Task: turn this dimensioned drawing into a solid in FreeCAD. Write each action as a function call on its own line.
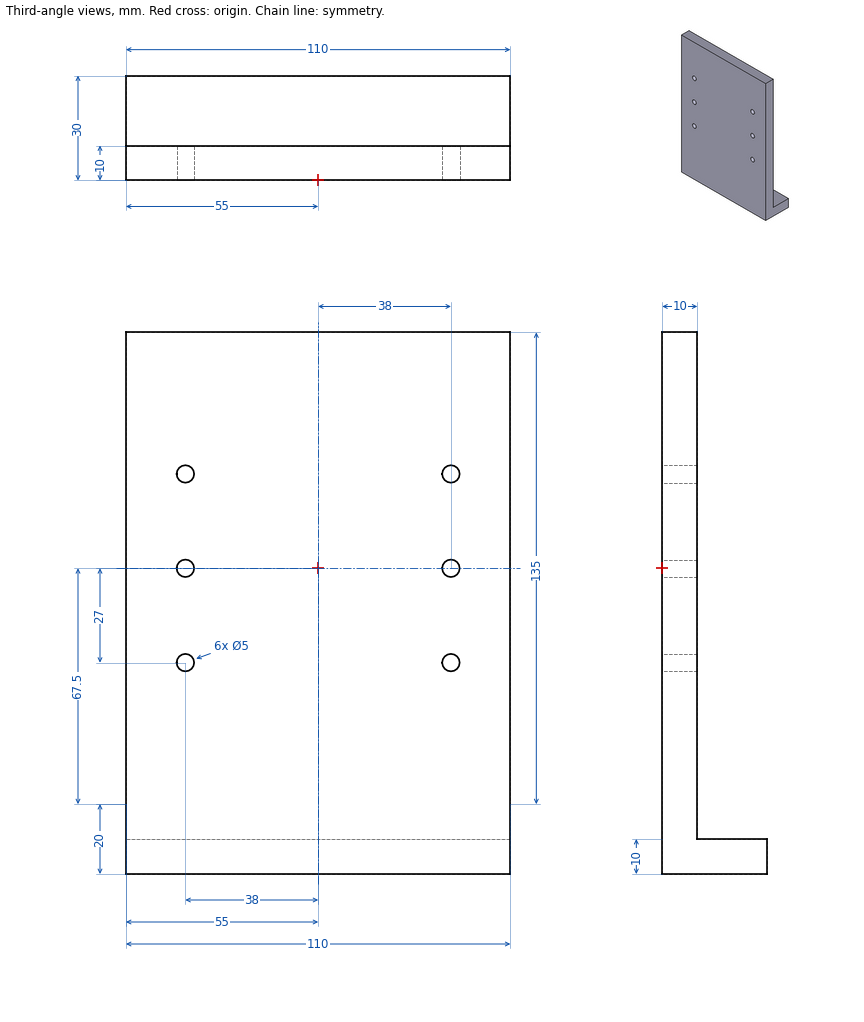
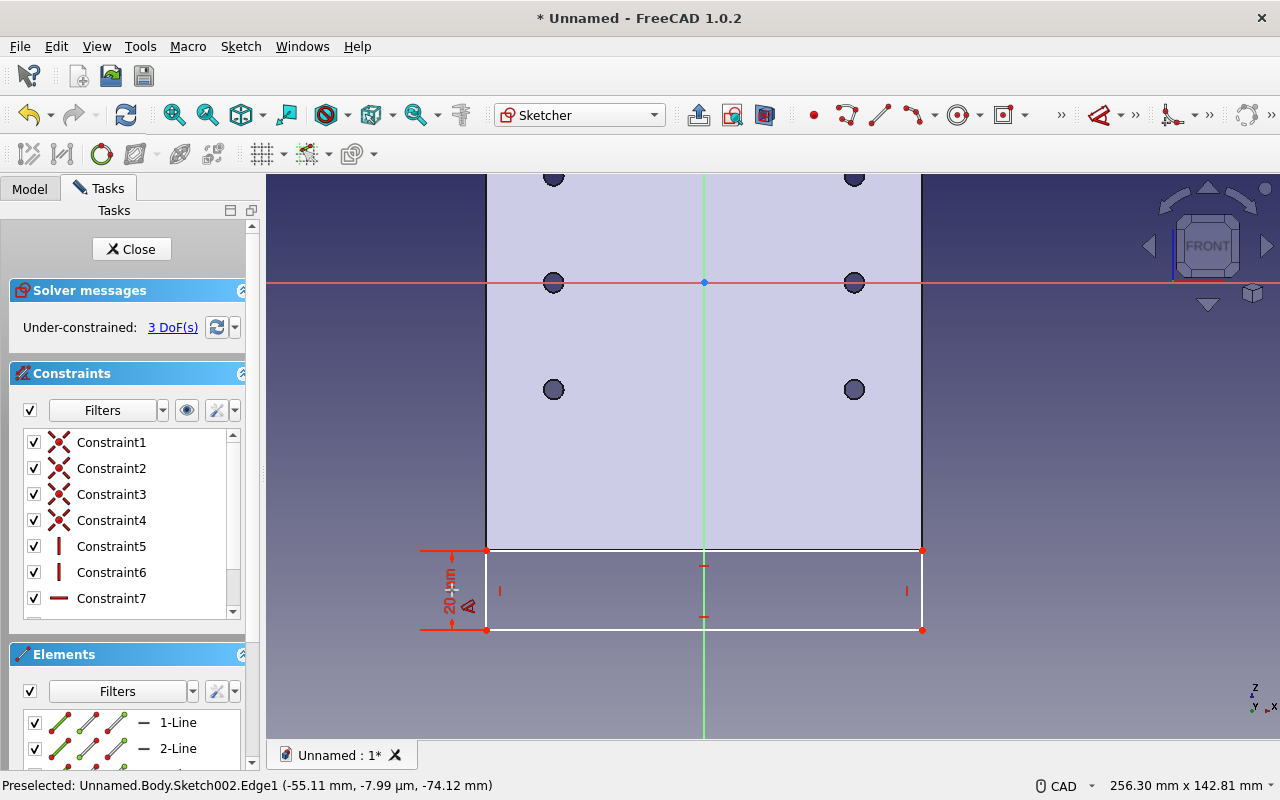
click(617, 630)
click(604, 664)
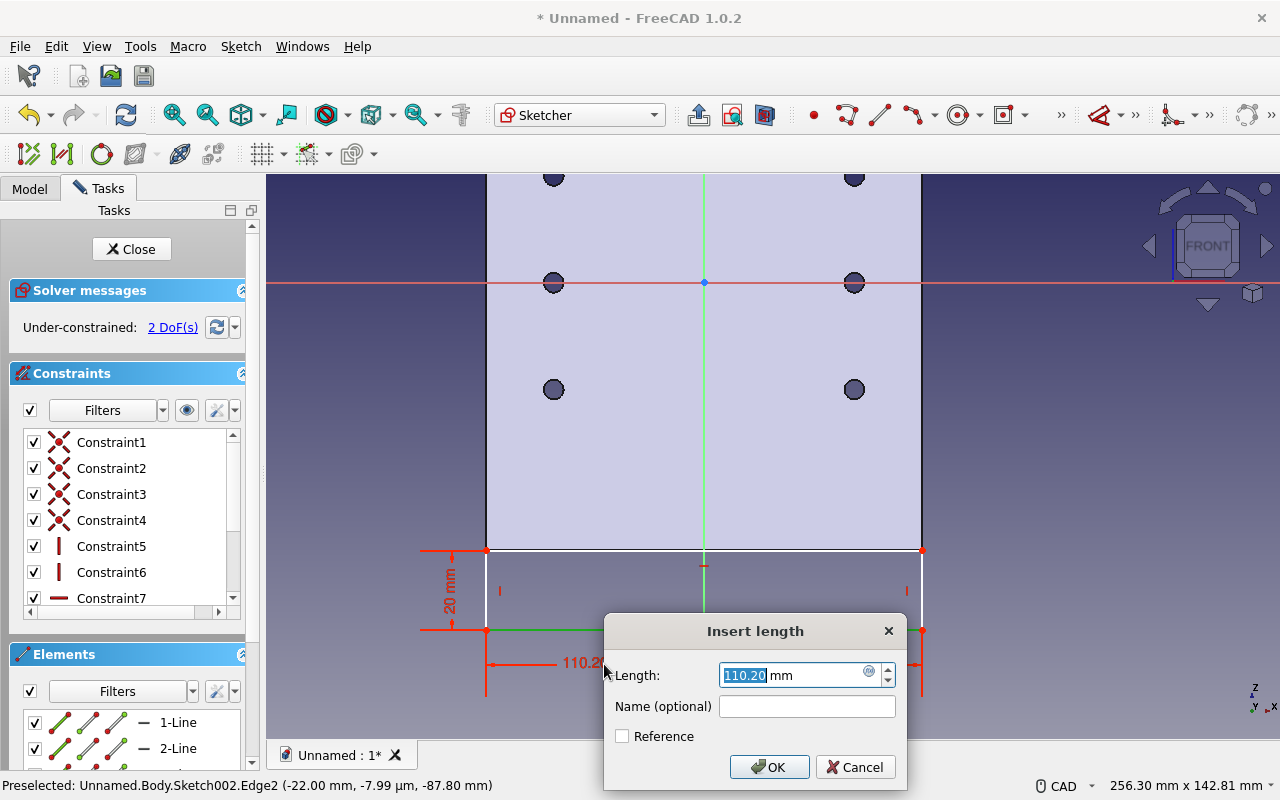
text(110)
key(Return)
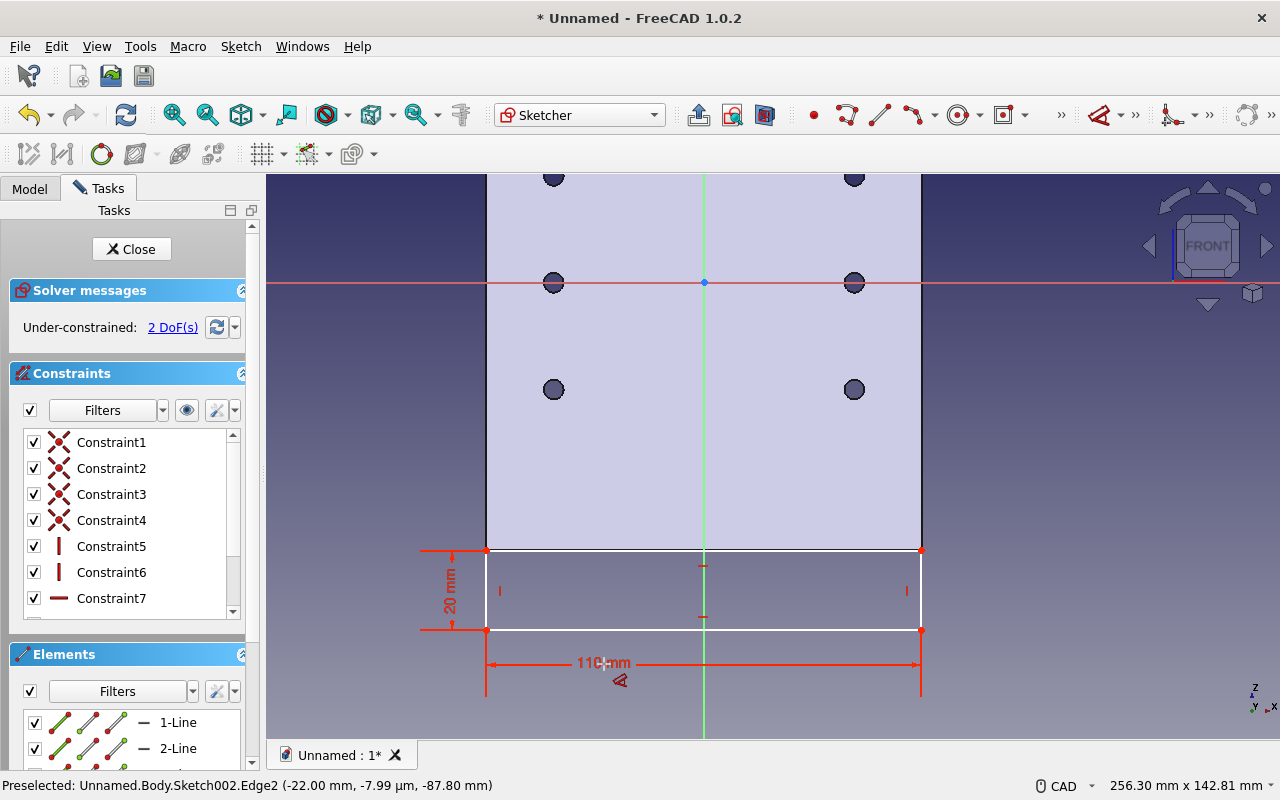
click(486, 551)
click(595, 249)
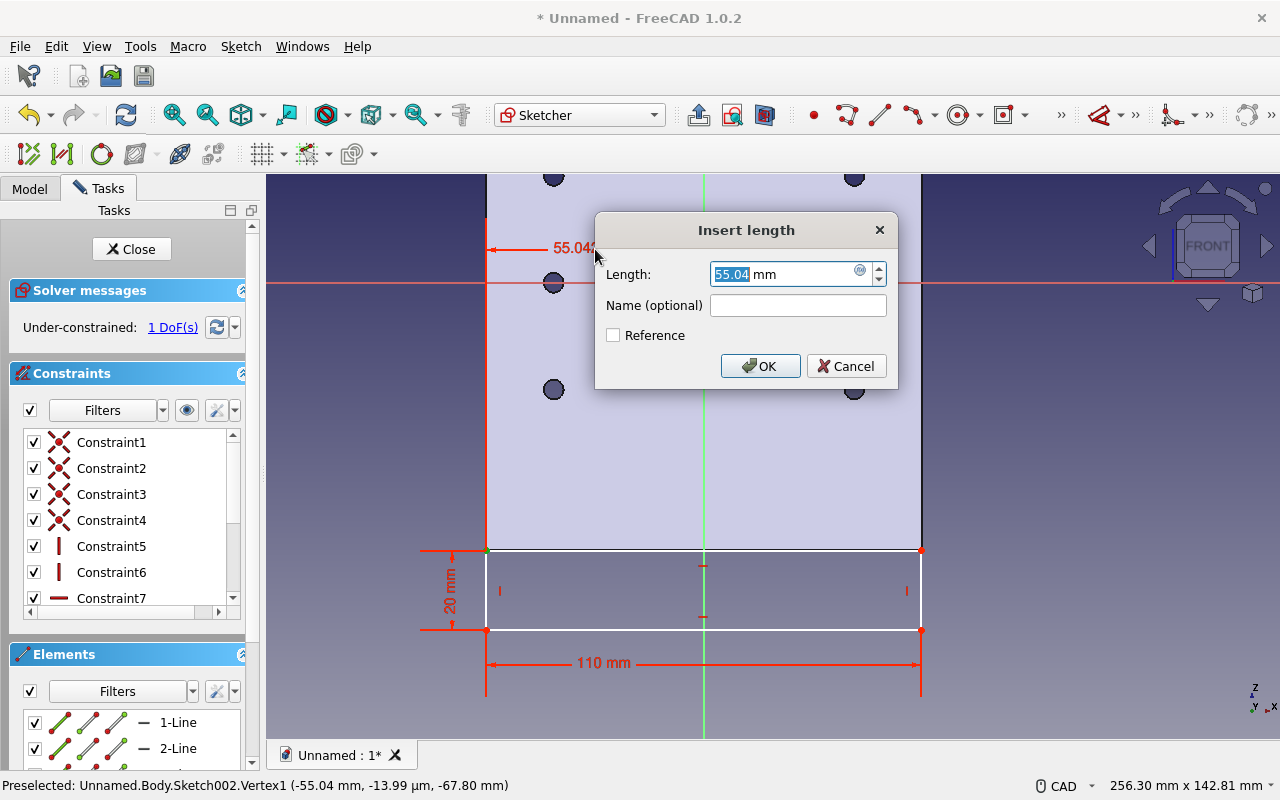
text(55)
key(Return)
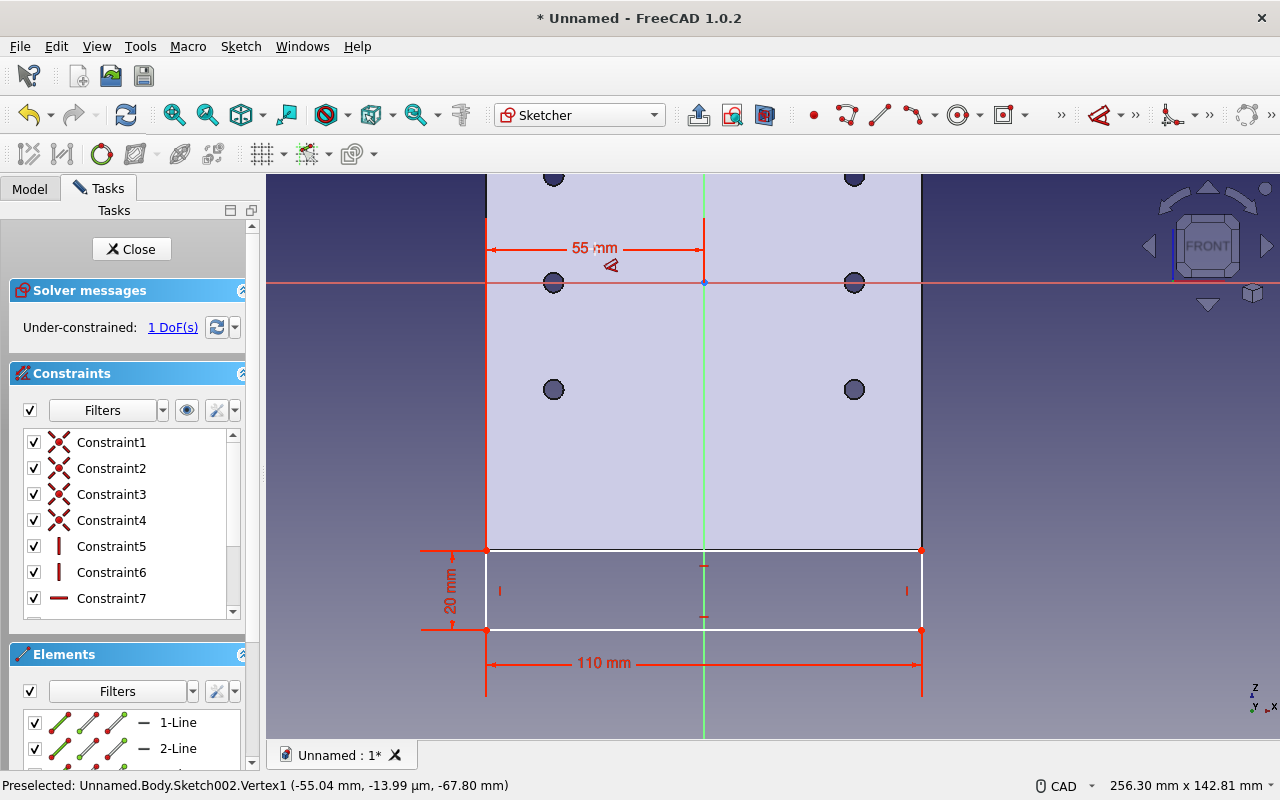
click(486, 551)
click(452, 417)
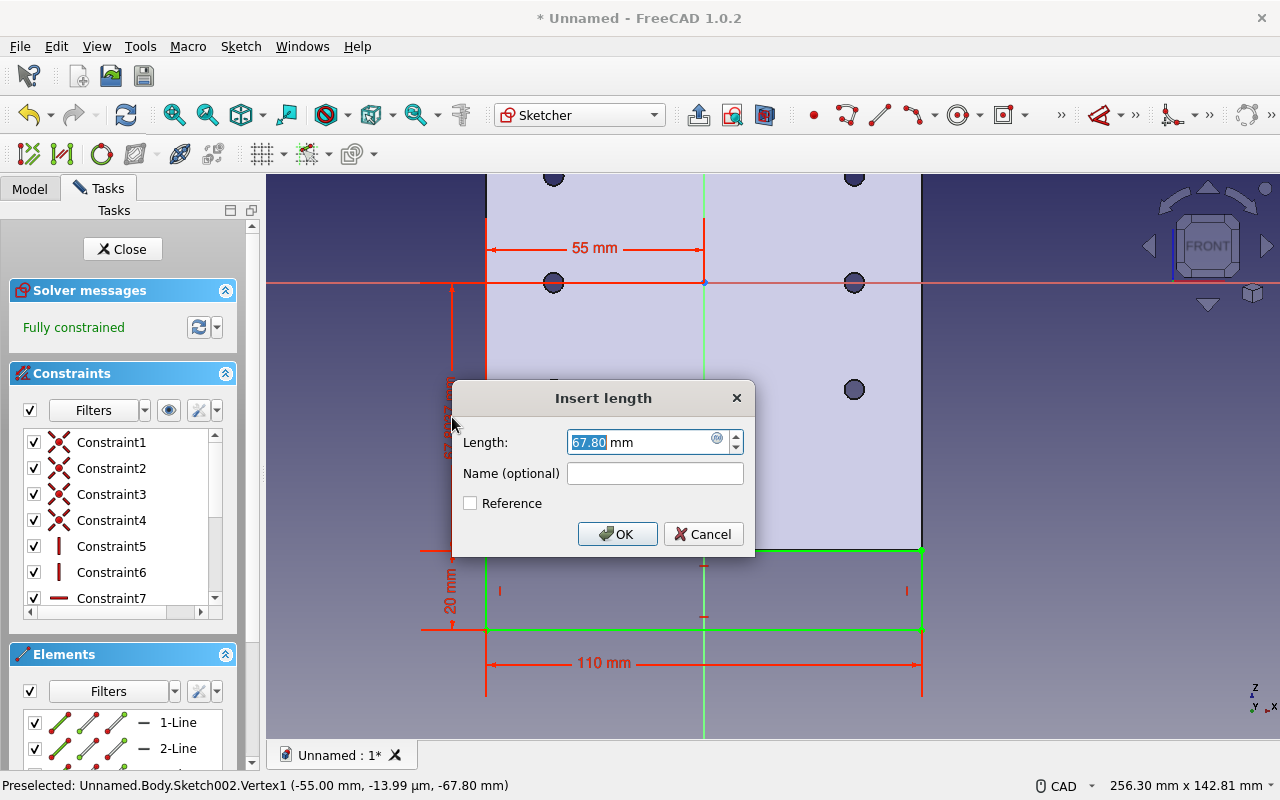
text(67.5)
key(Return)
key(Escape)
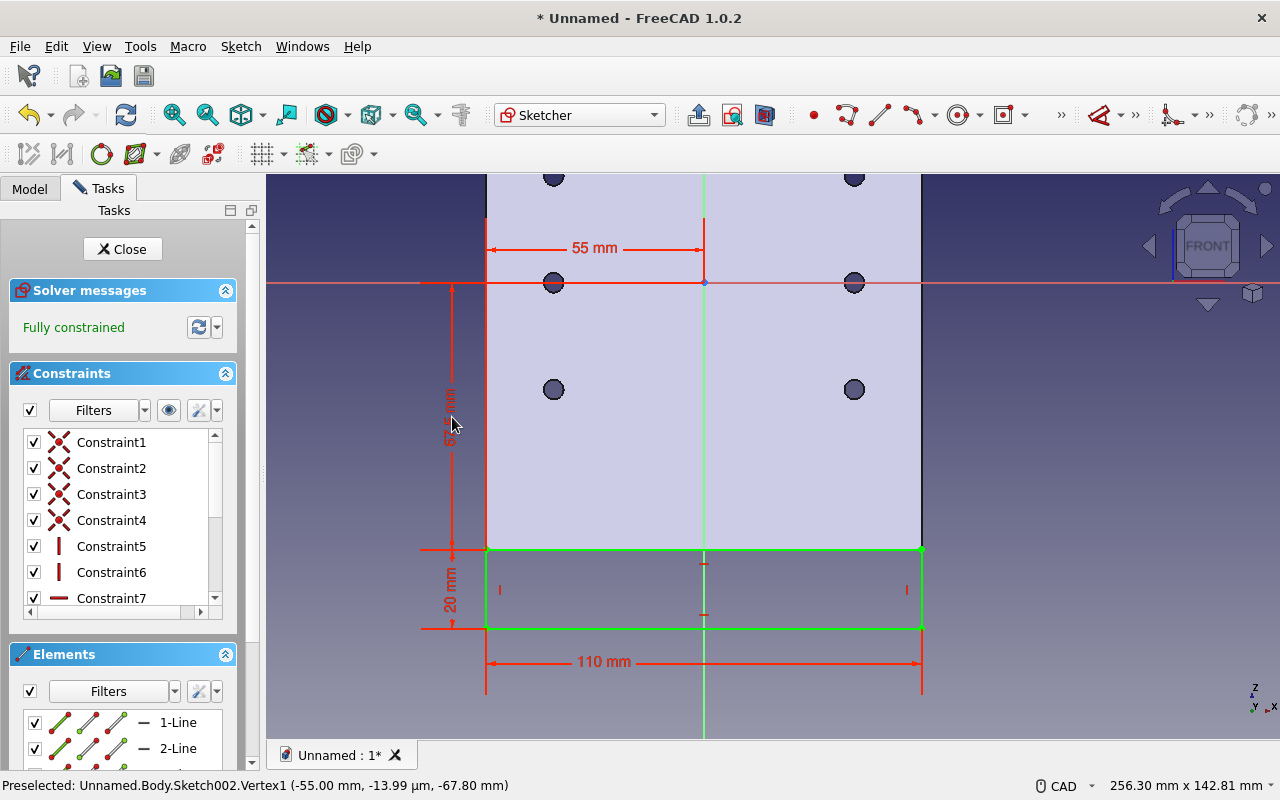
click(123, 249)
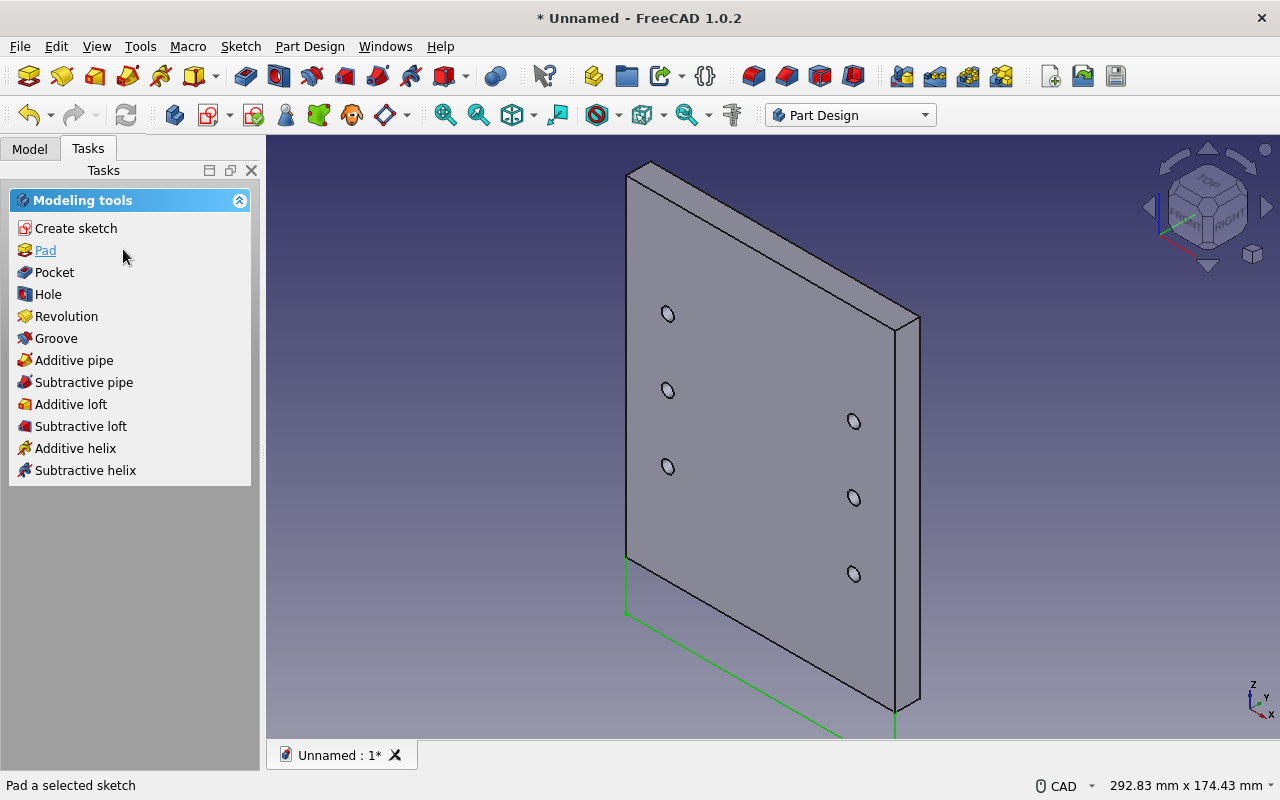
click(29, 76)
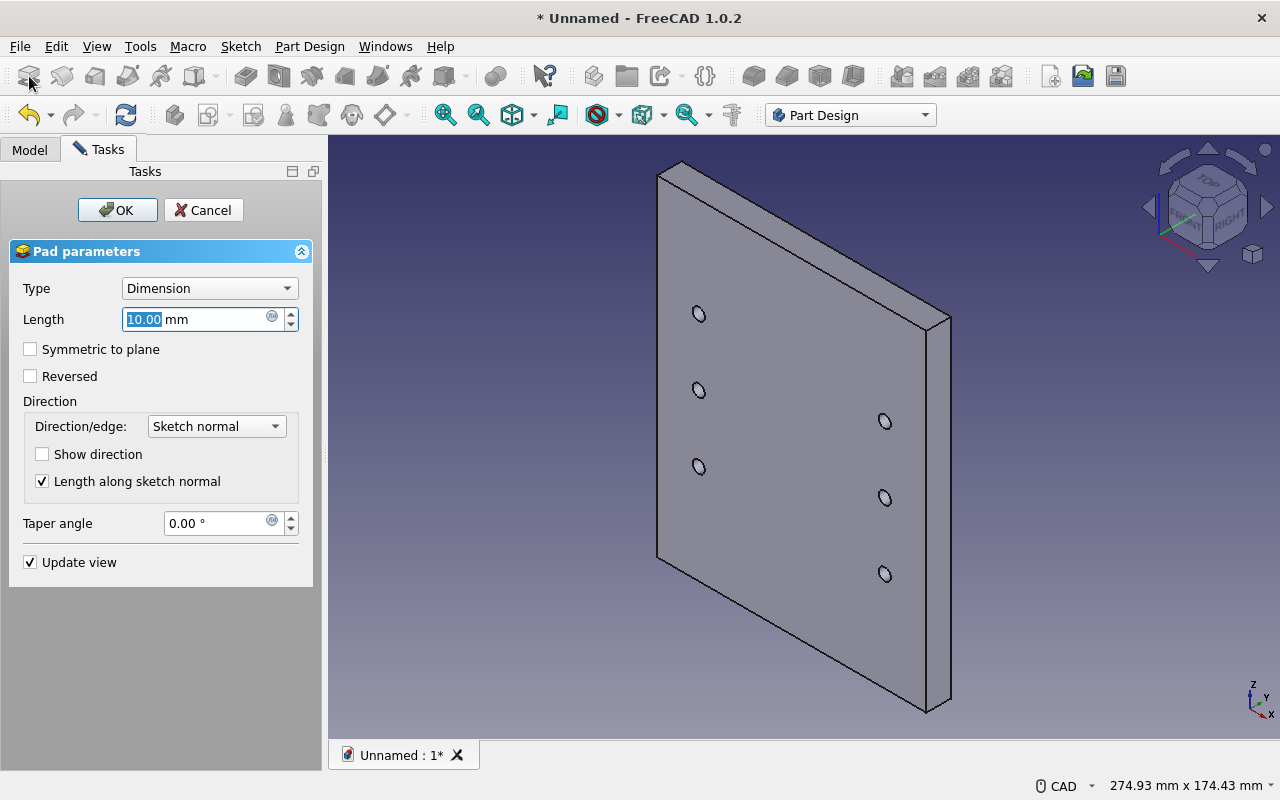
text(10)
key(Tab)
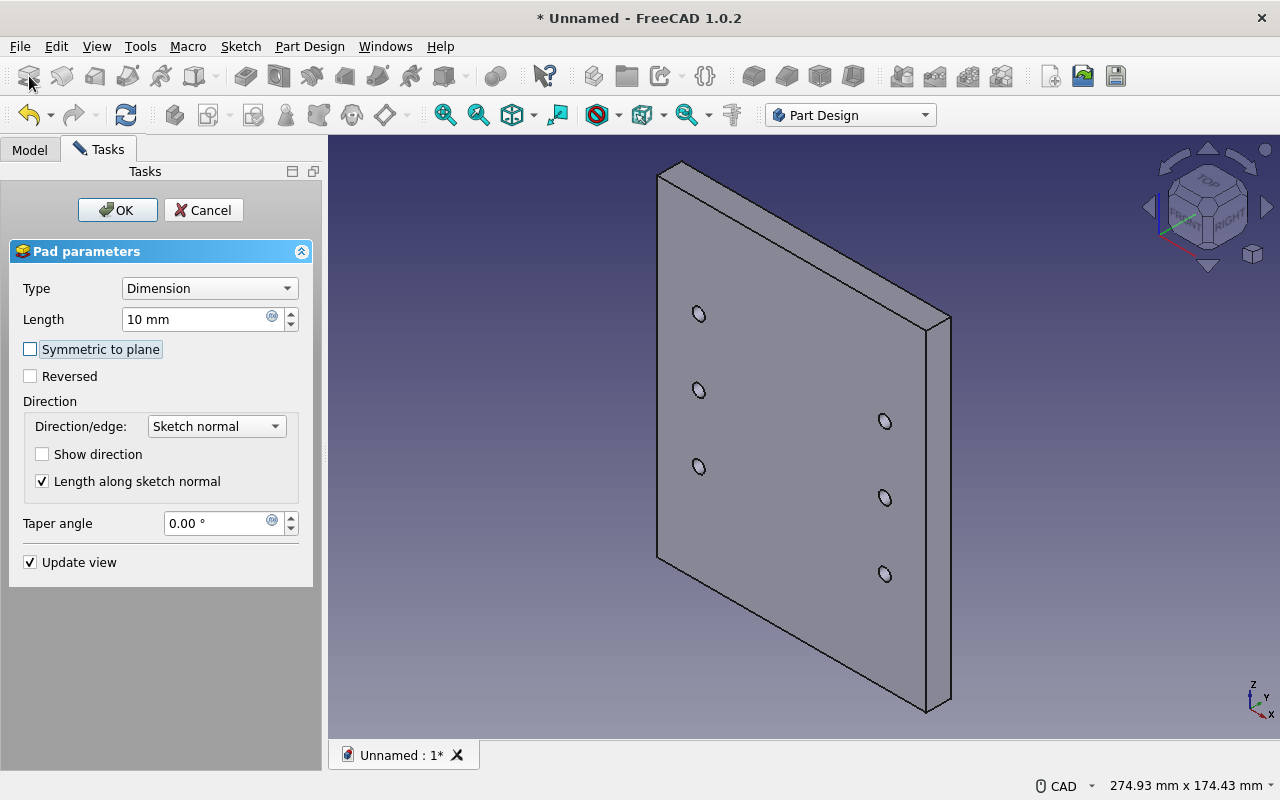
click(31, 376)